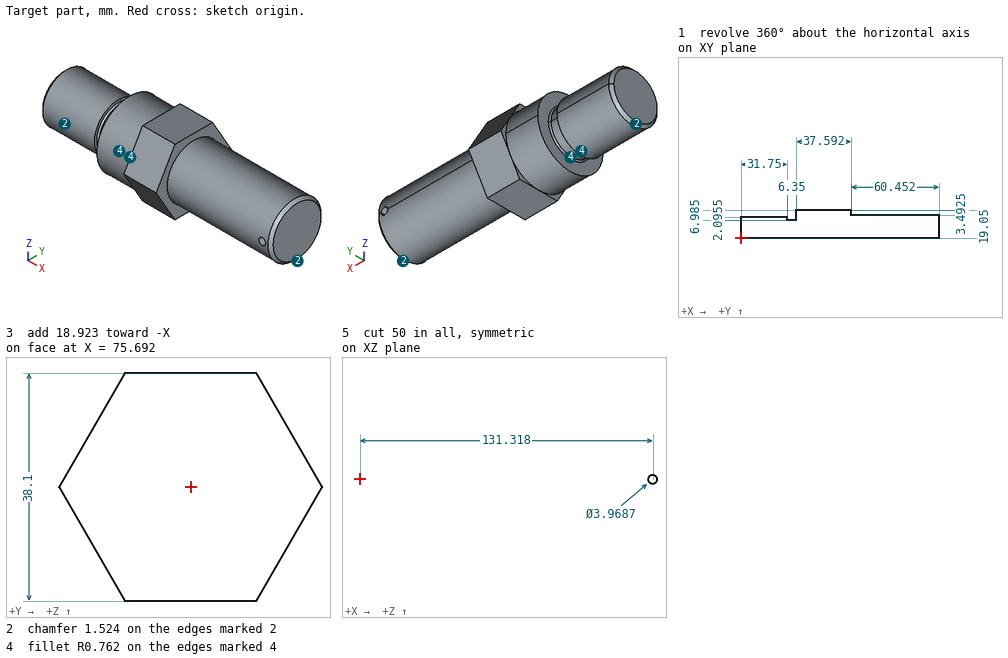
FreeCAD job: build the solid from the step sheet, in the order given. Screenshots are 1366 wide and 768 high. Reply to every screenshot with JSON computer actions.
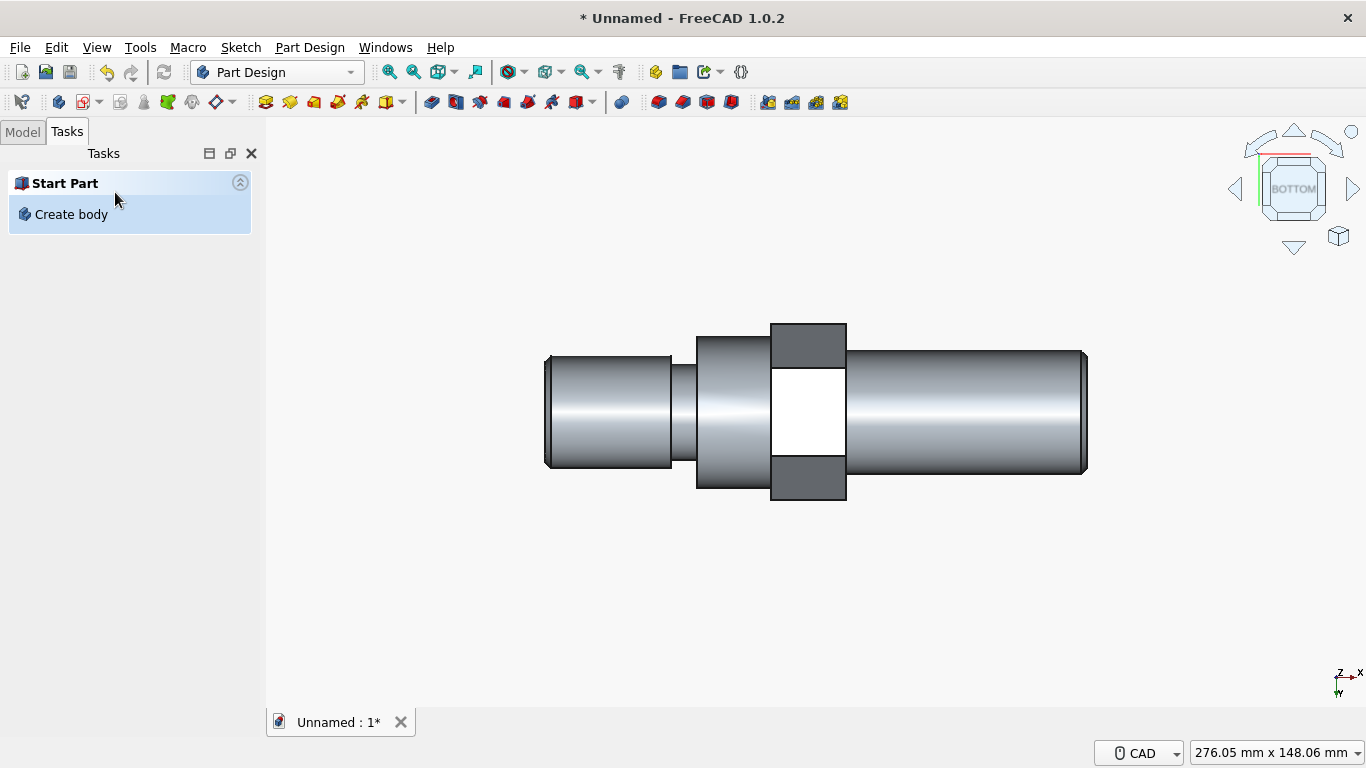
{"action": "key", "text": "4"}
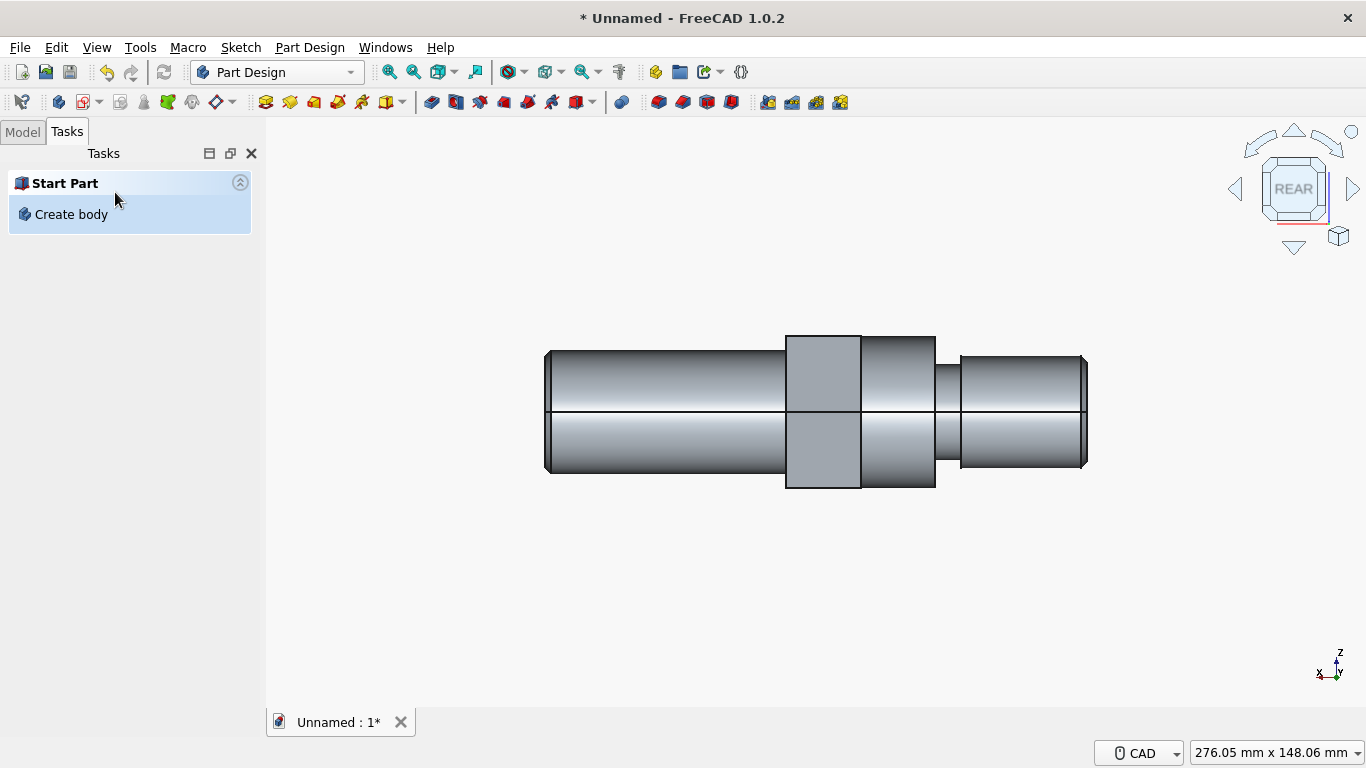
{"action": "key", "text": "6"}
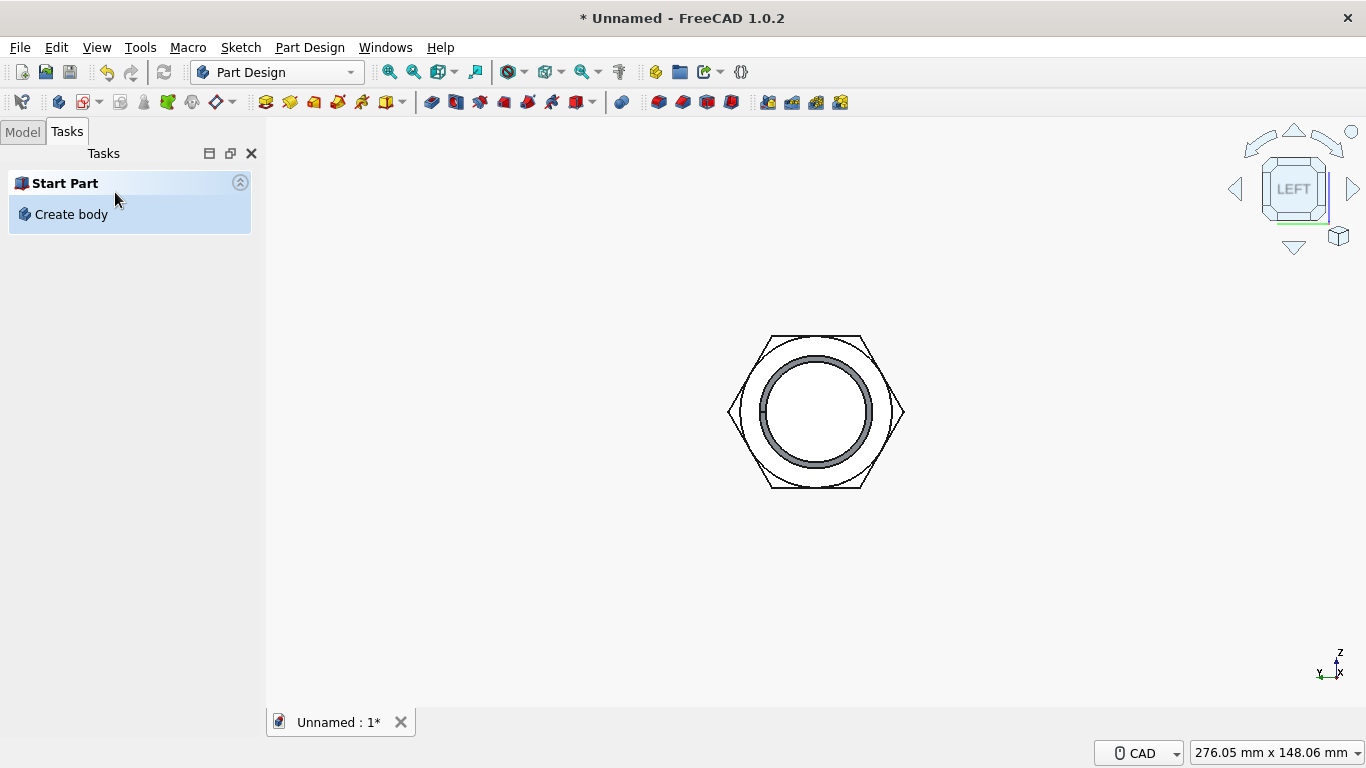
{"action": "key", "text": "v f"}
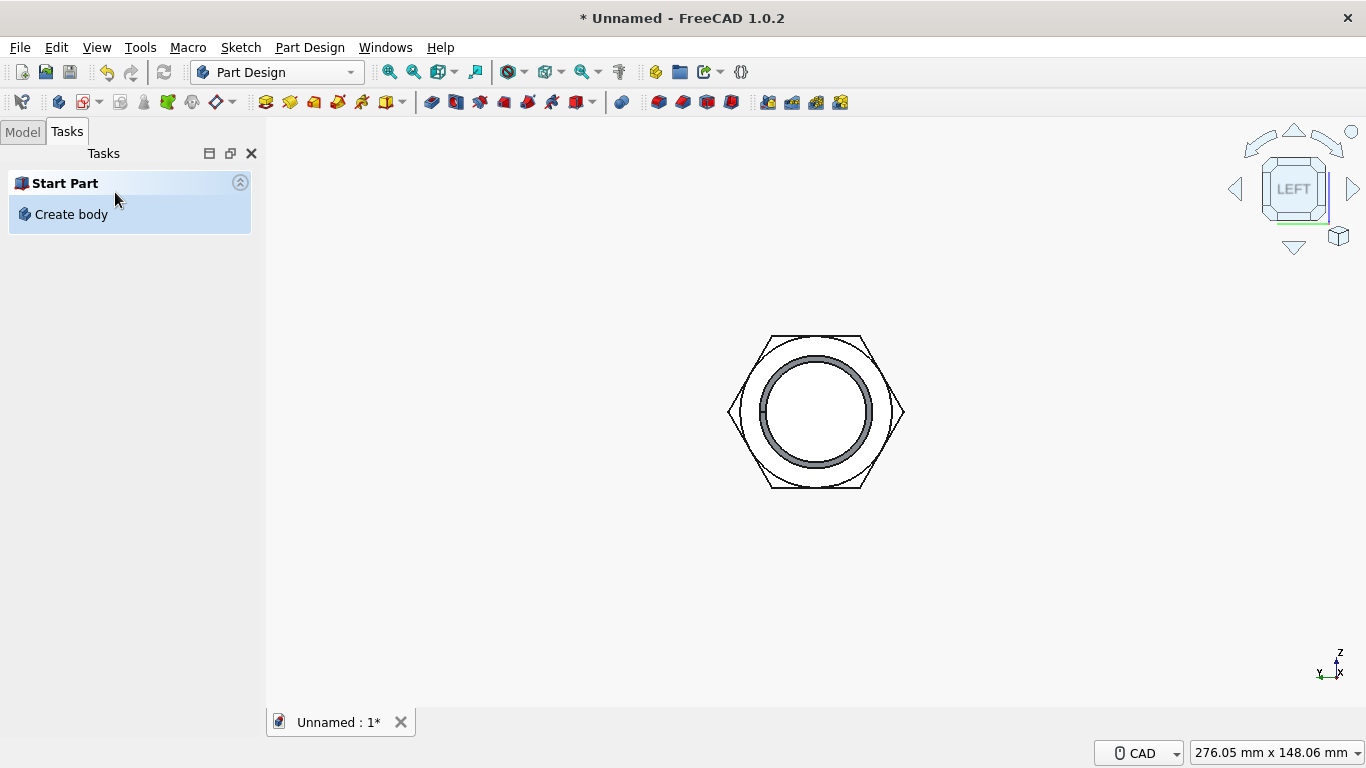
{"action": "key", "text": "v 3"}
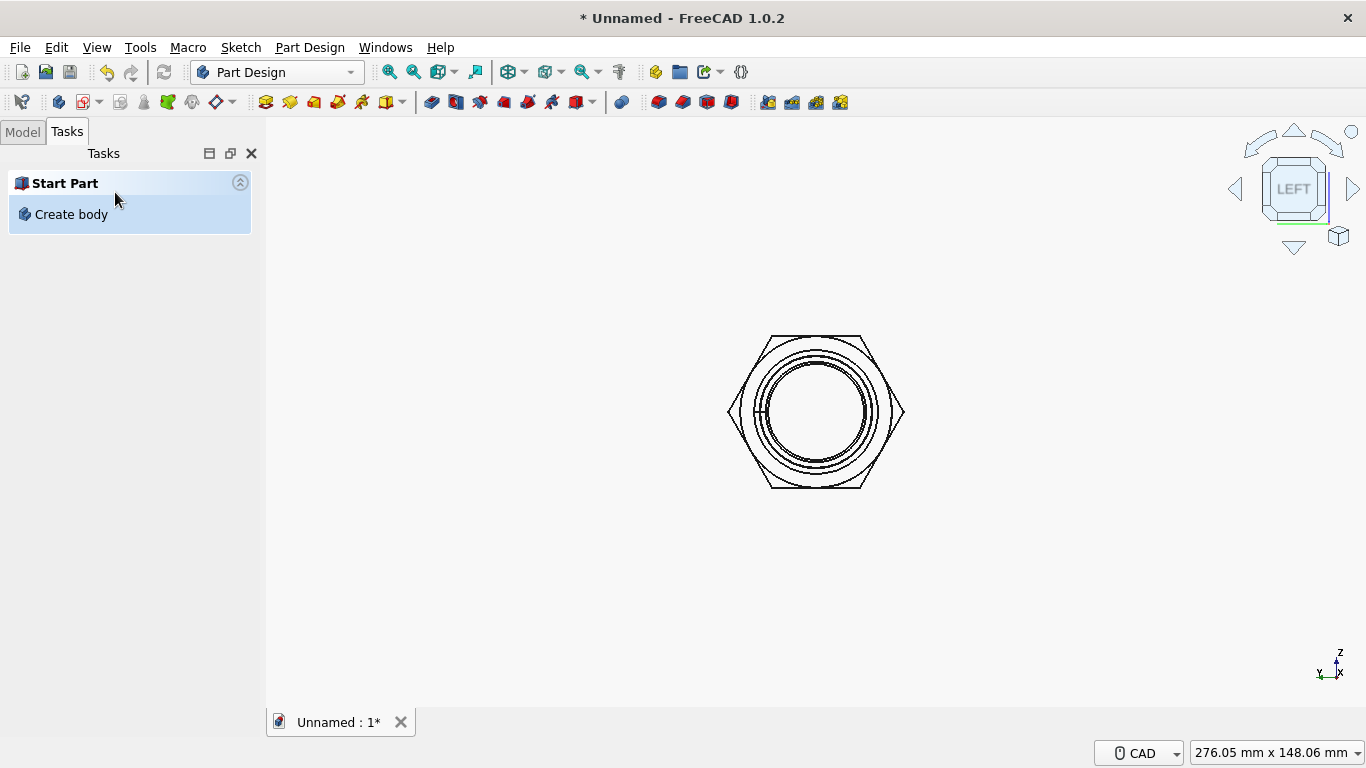
{"action": "key", "text": "0"}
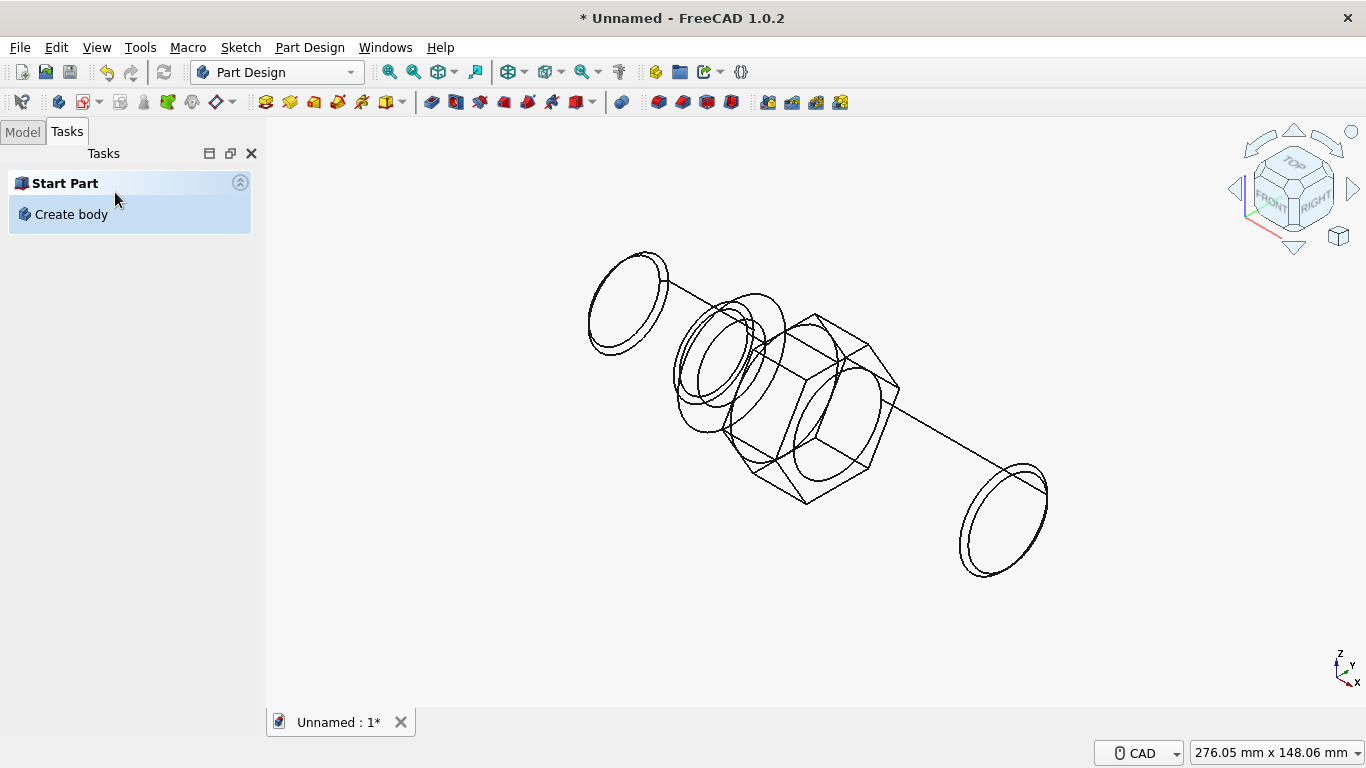
{"action": "left_click", "coordinate": [698, 382]}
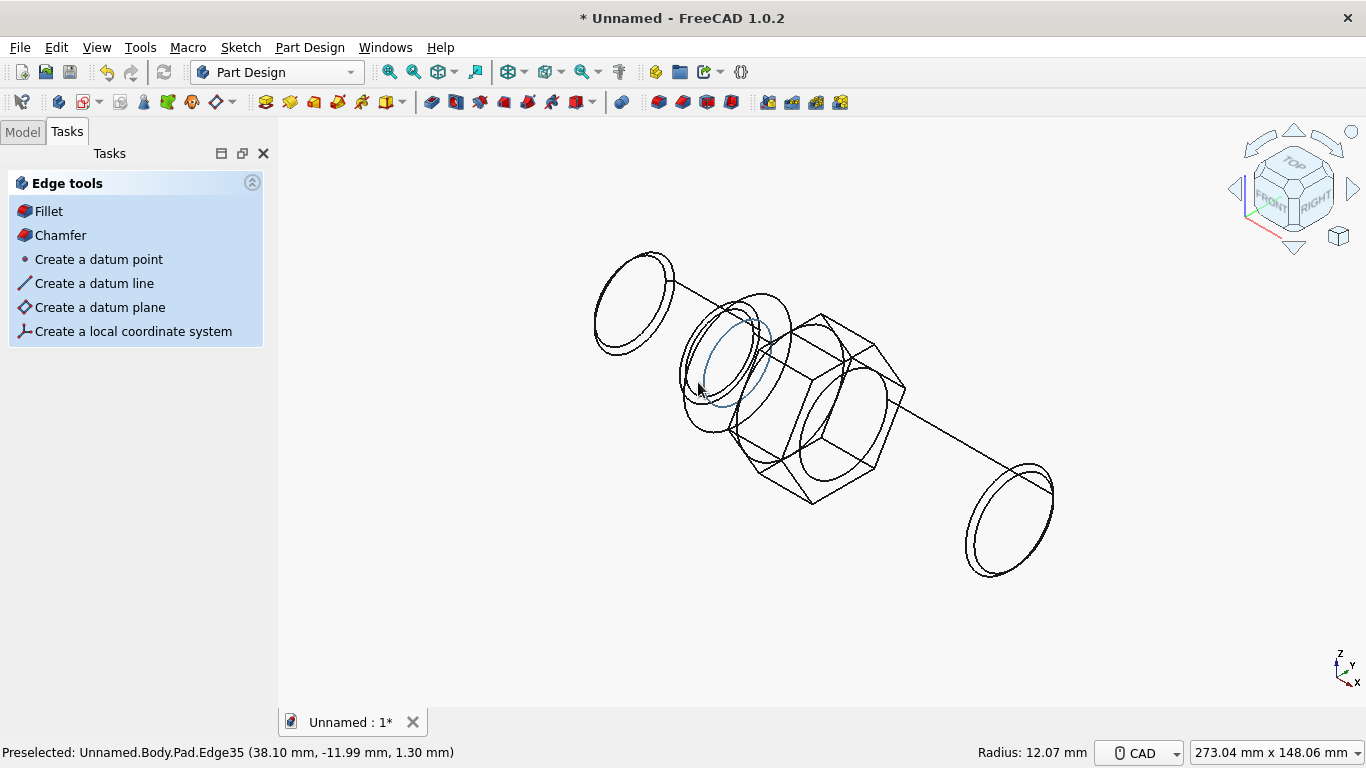
{"action": "left_click", "coordinate": [692, 391], "text": "ctrl"}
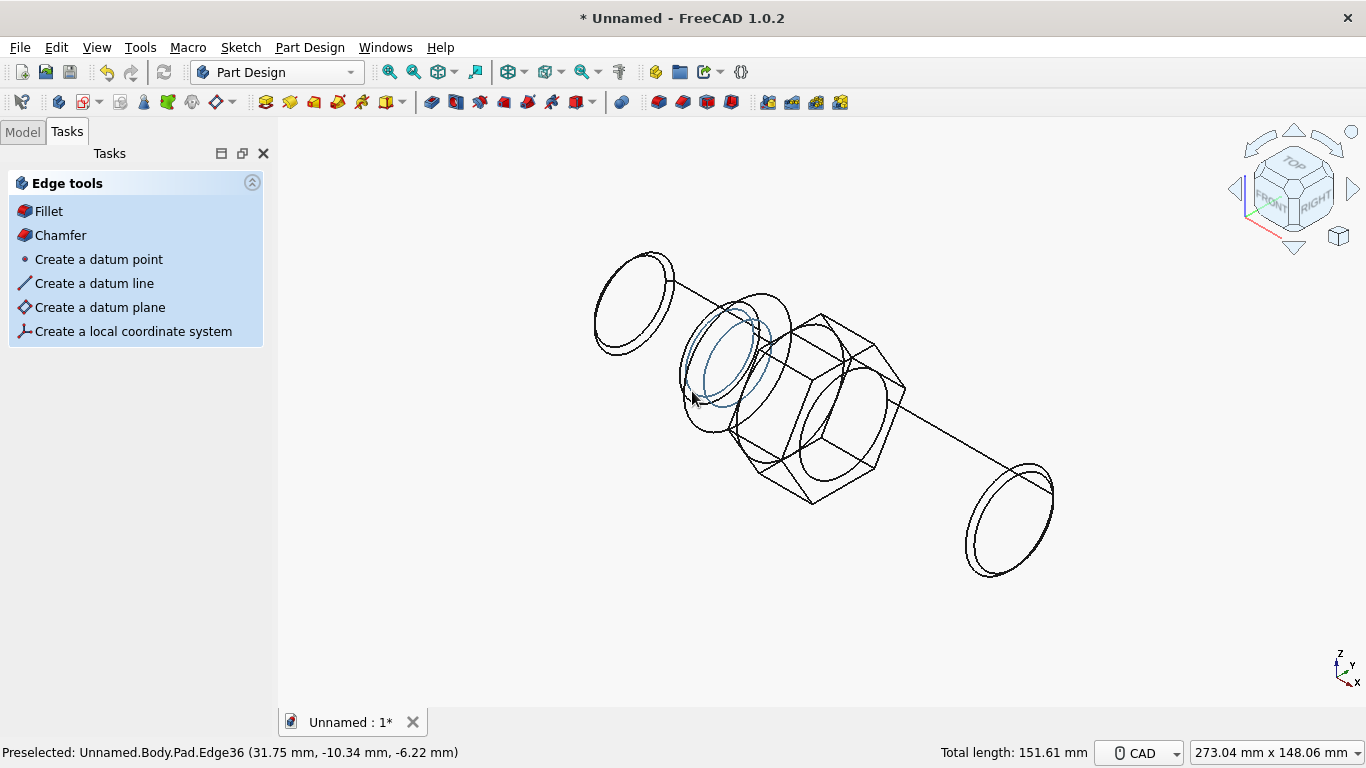
{"action": "key", "text": "v 1"}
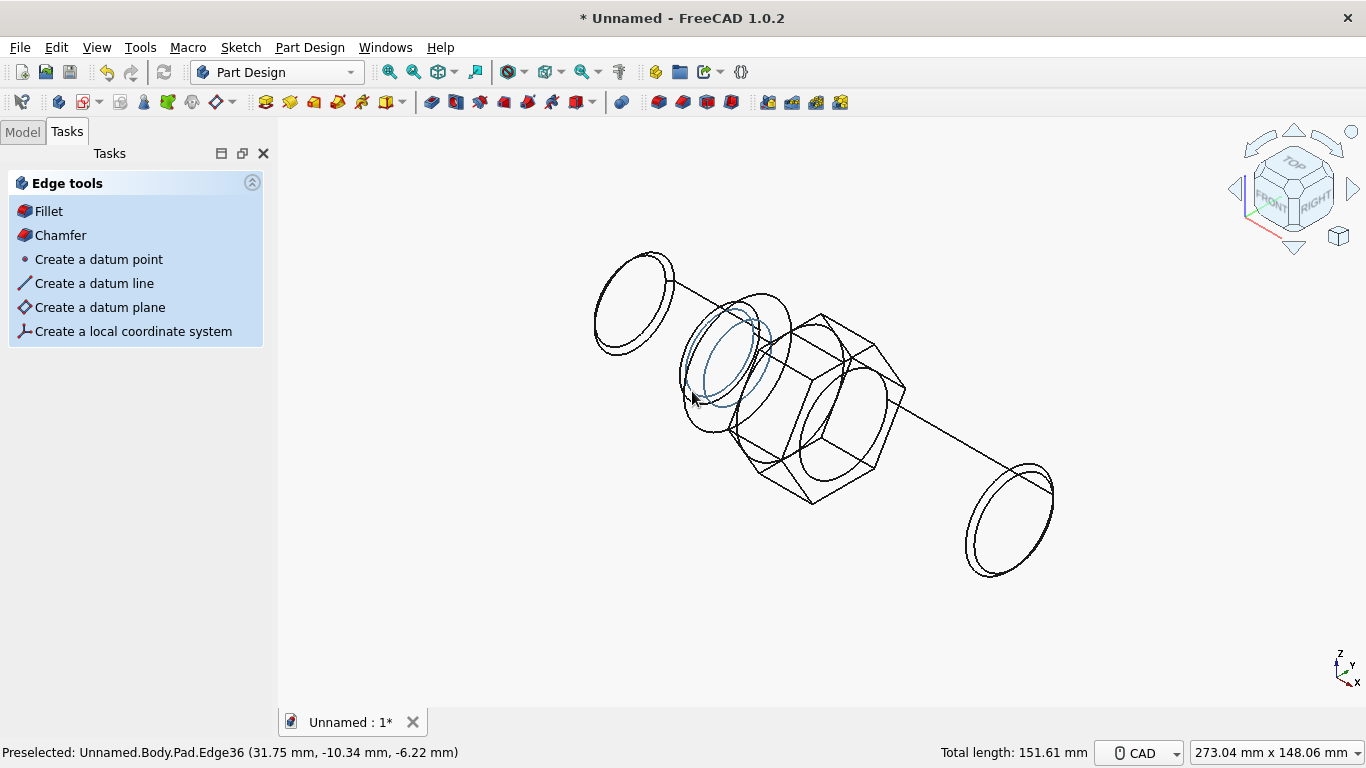
{"action": "left_click", "coordinate": [660, 102]}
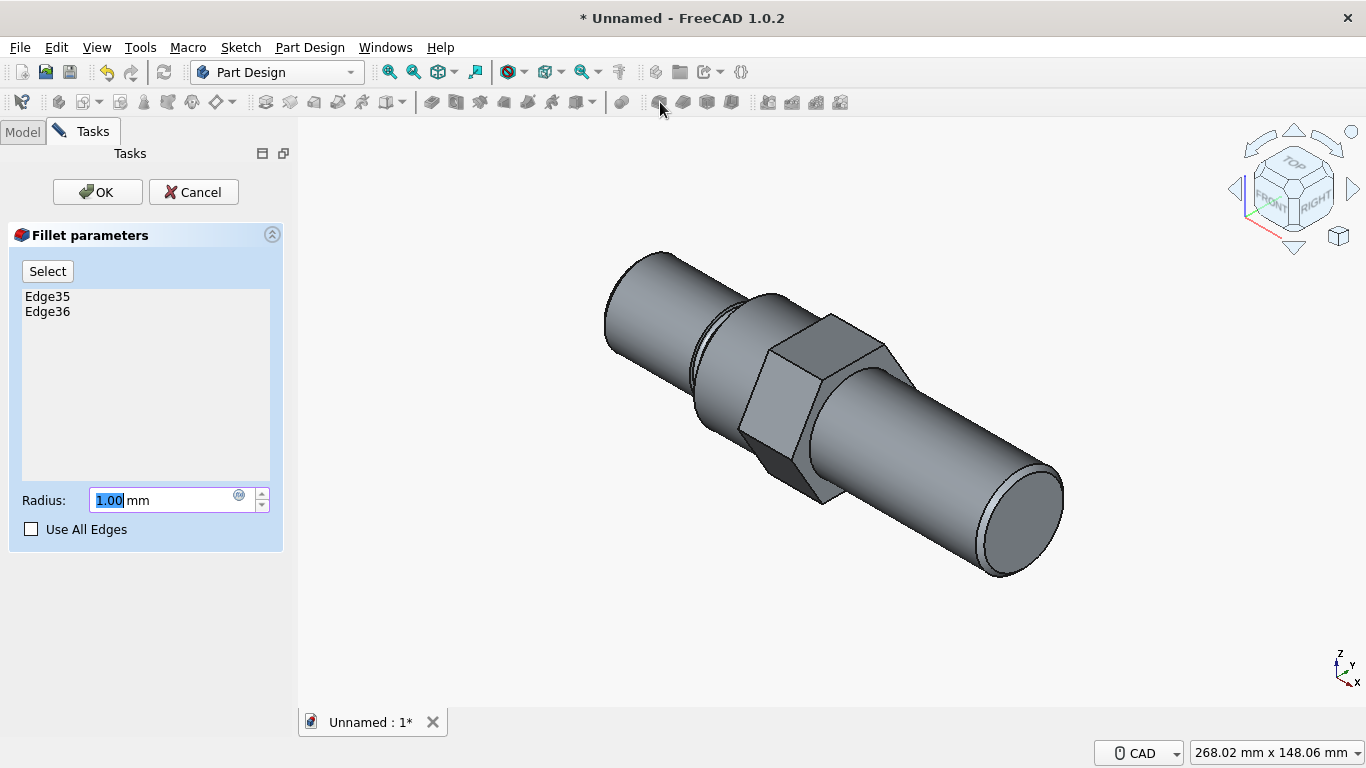
{"action": "type", "text": "0.762"}
{"action": "key", "text": "Tab"}